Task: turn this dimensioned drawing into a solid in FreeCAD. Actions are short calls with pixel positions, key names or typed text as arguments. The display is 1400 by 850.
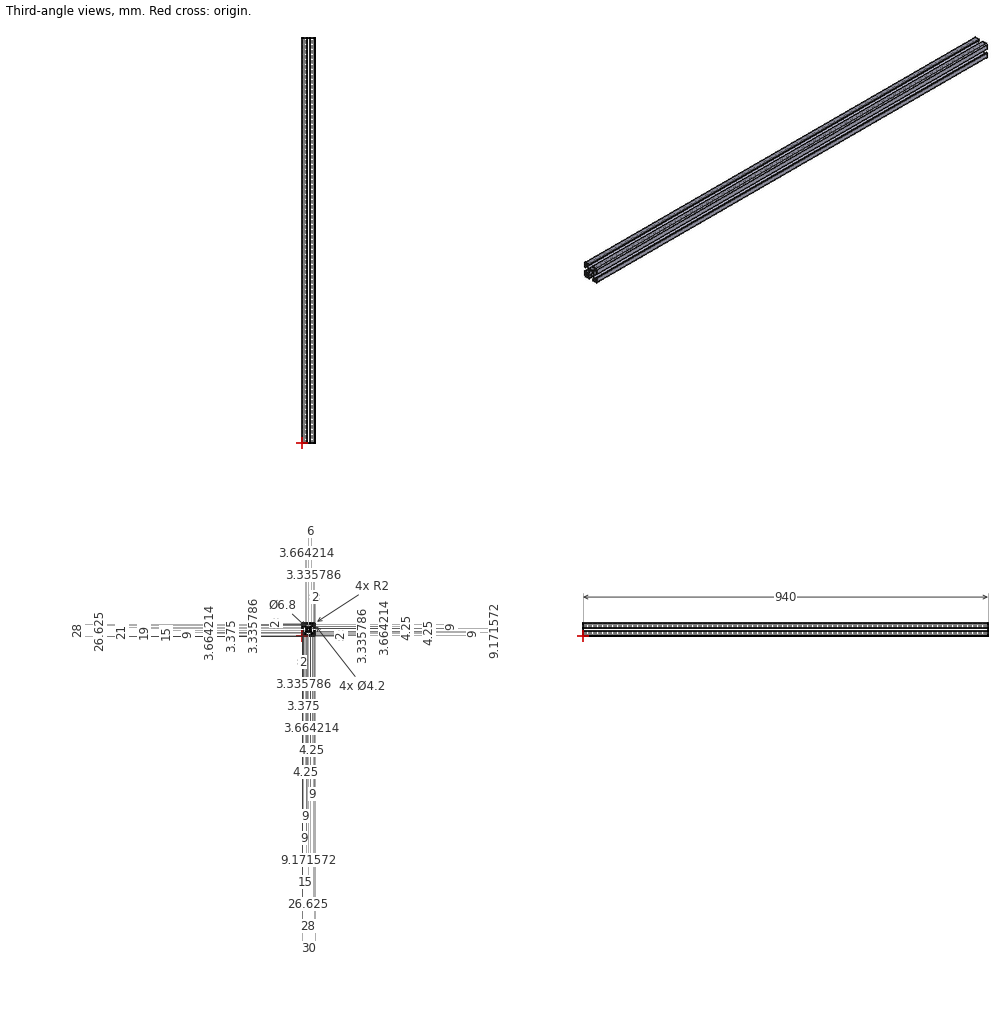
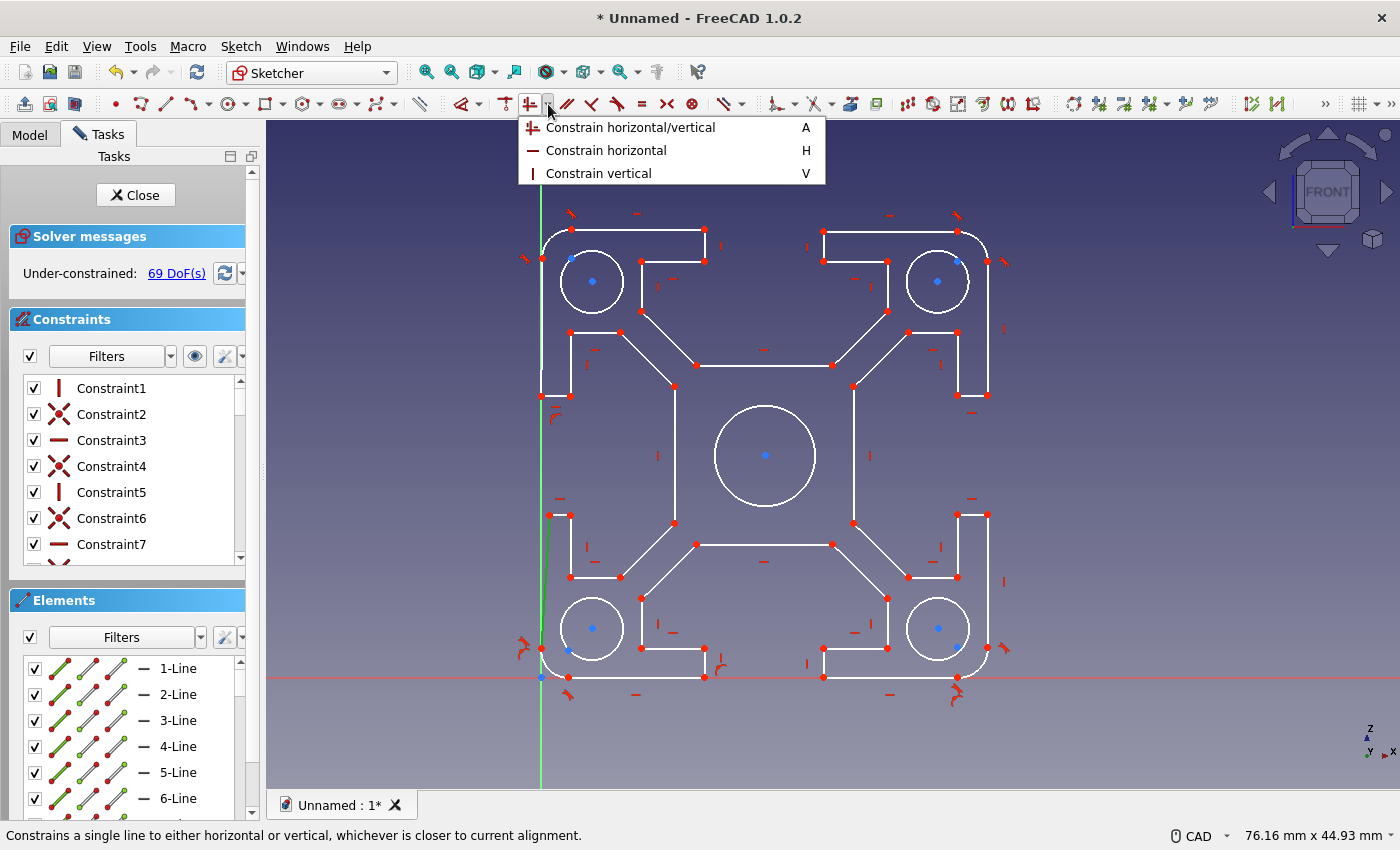
click(672, 174)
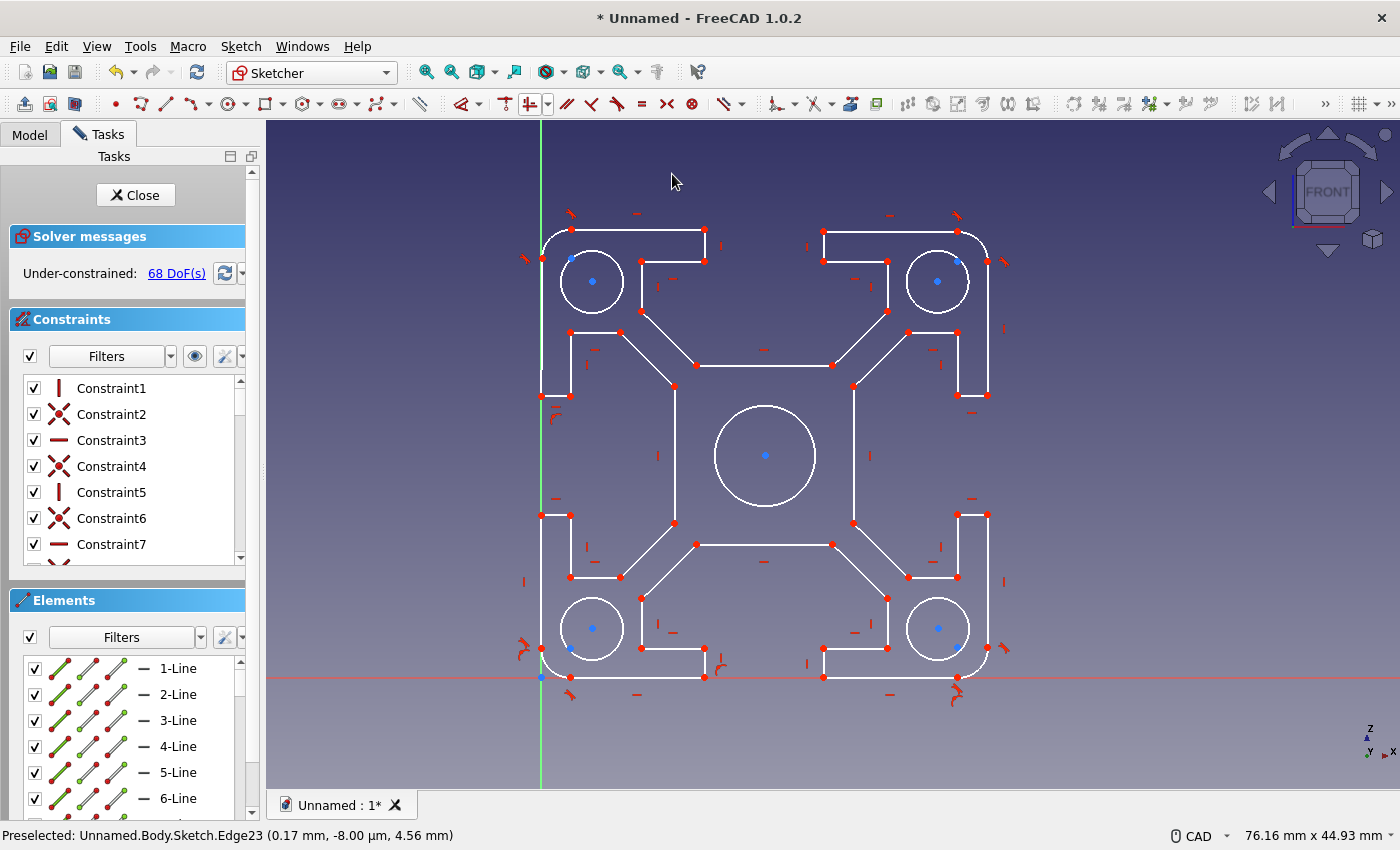
click(542, 355)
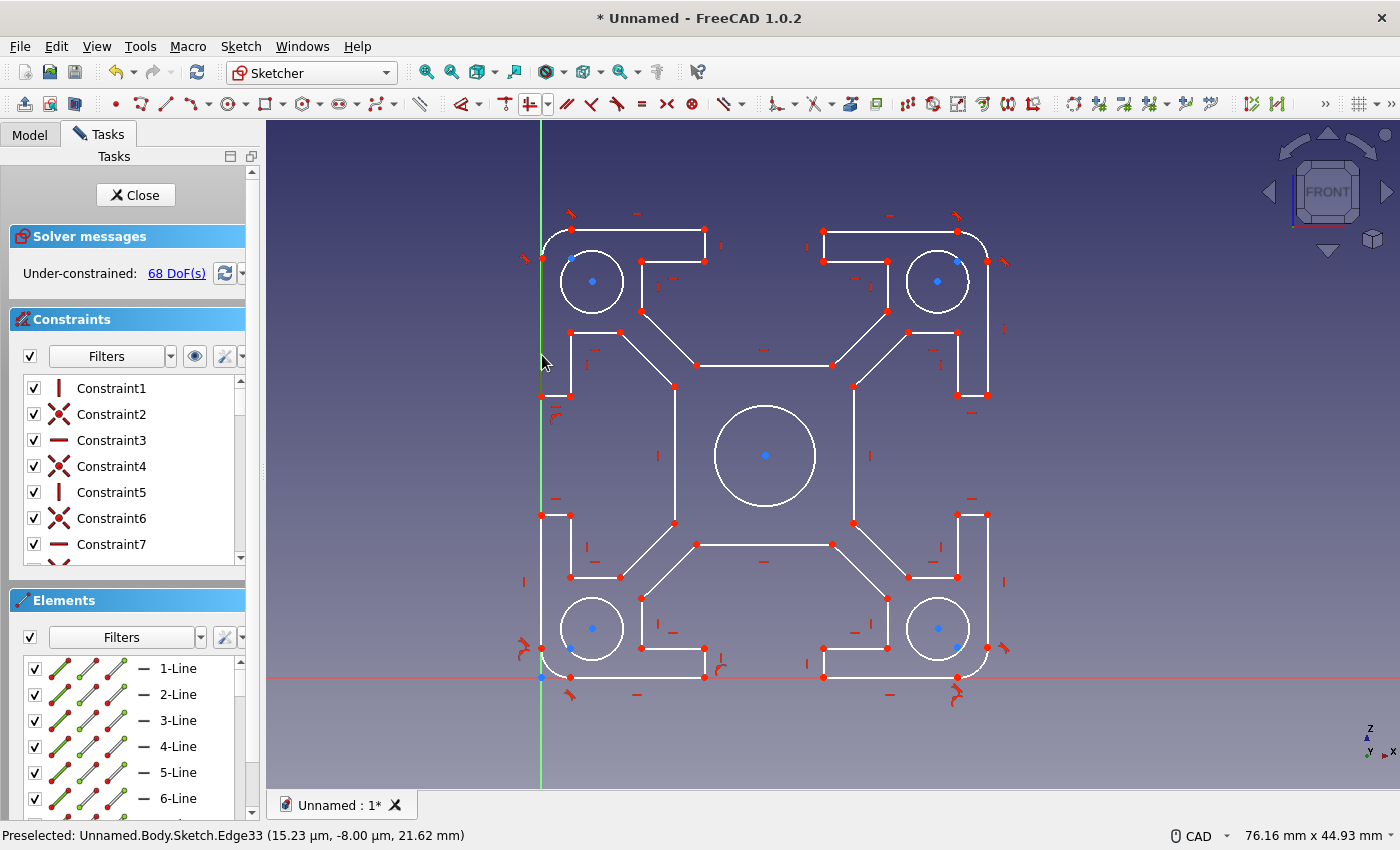
key(v)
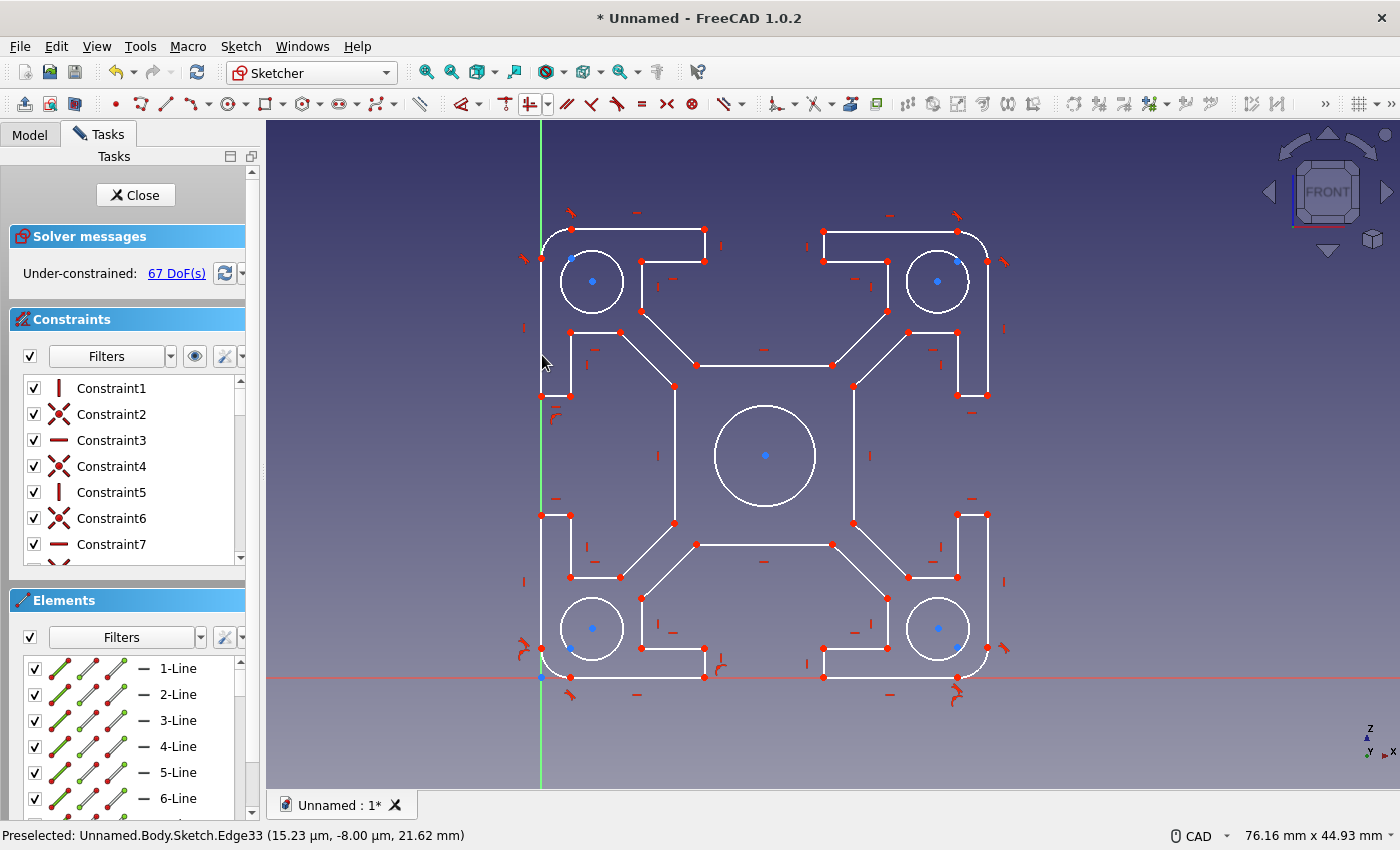
click(972, 675)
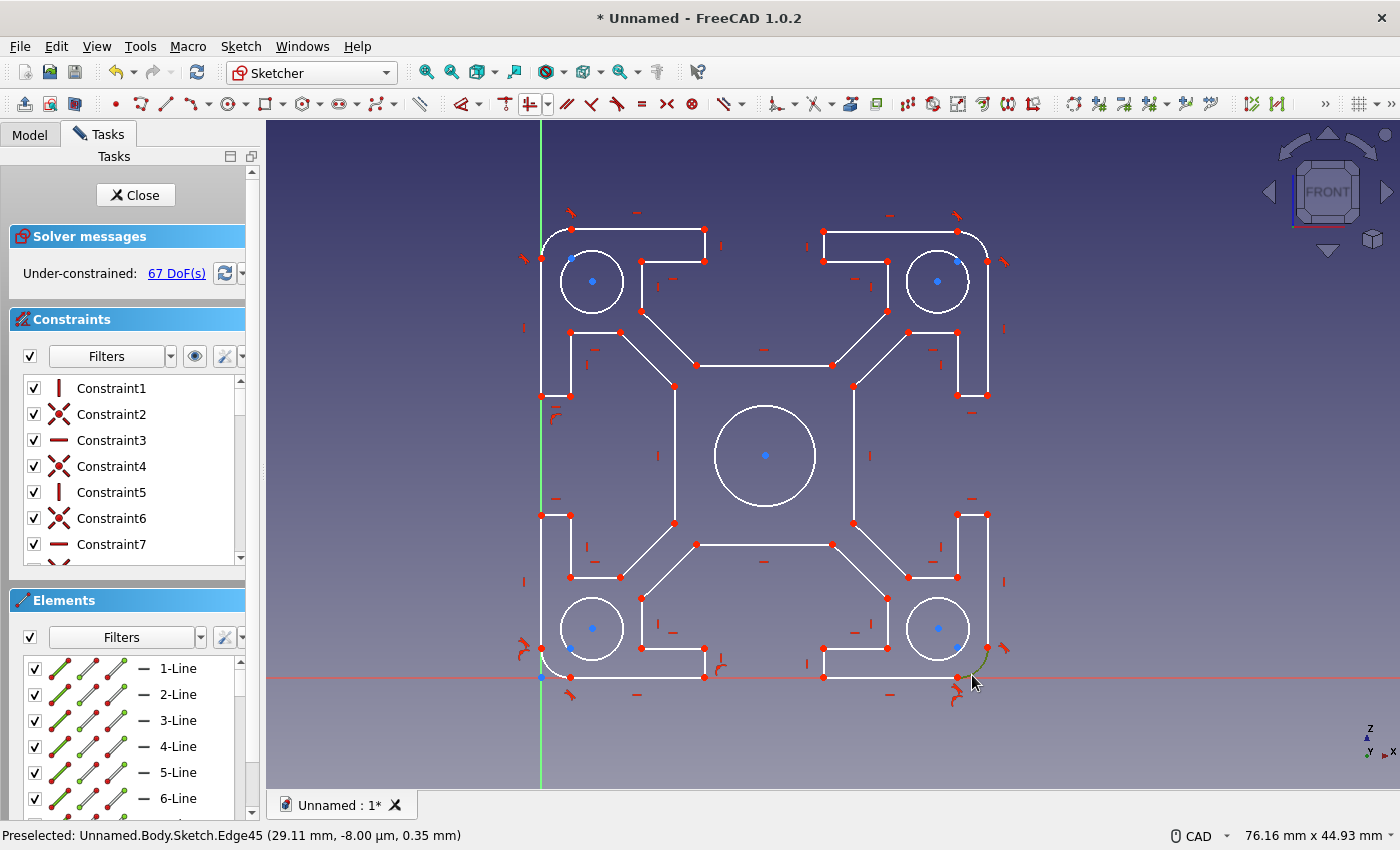
click(545, 662)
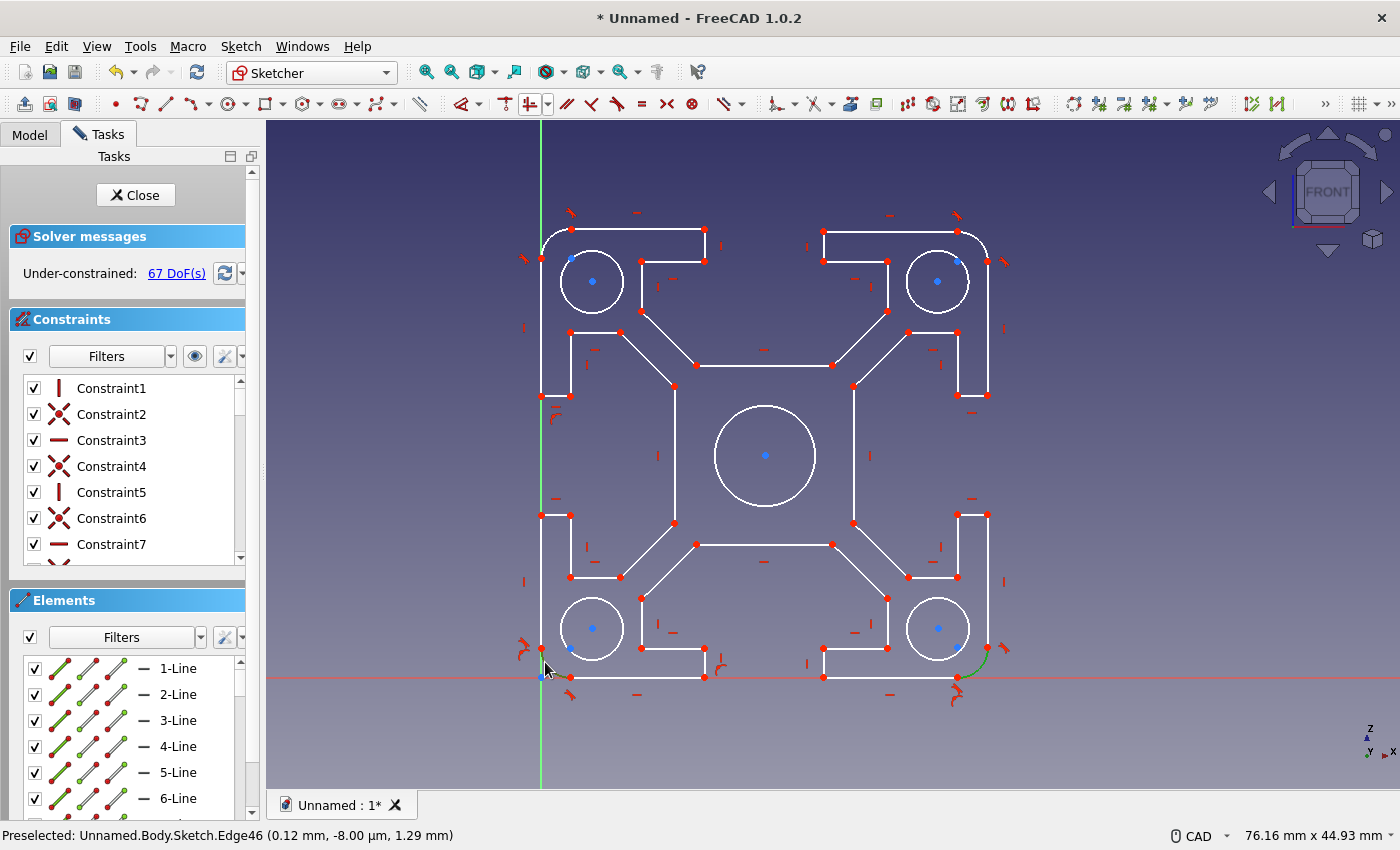
click(558, 232)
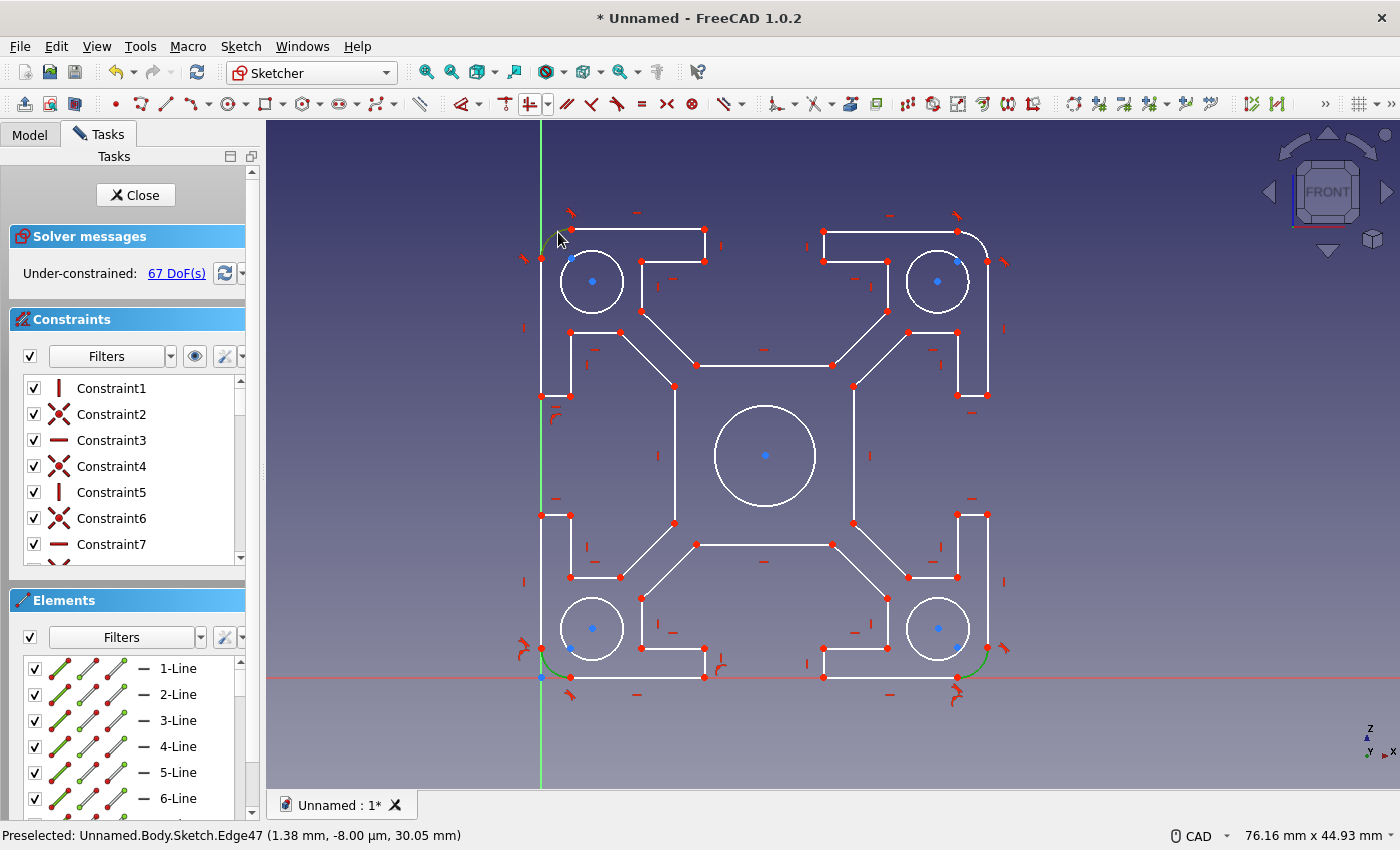
click(985, 248)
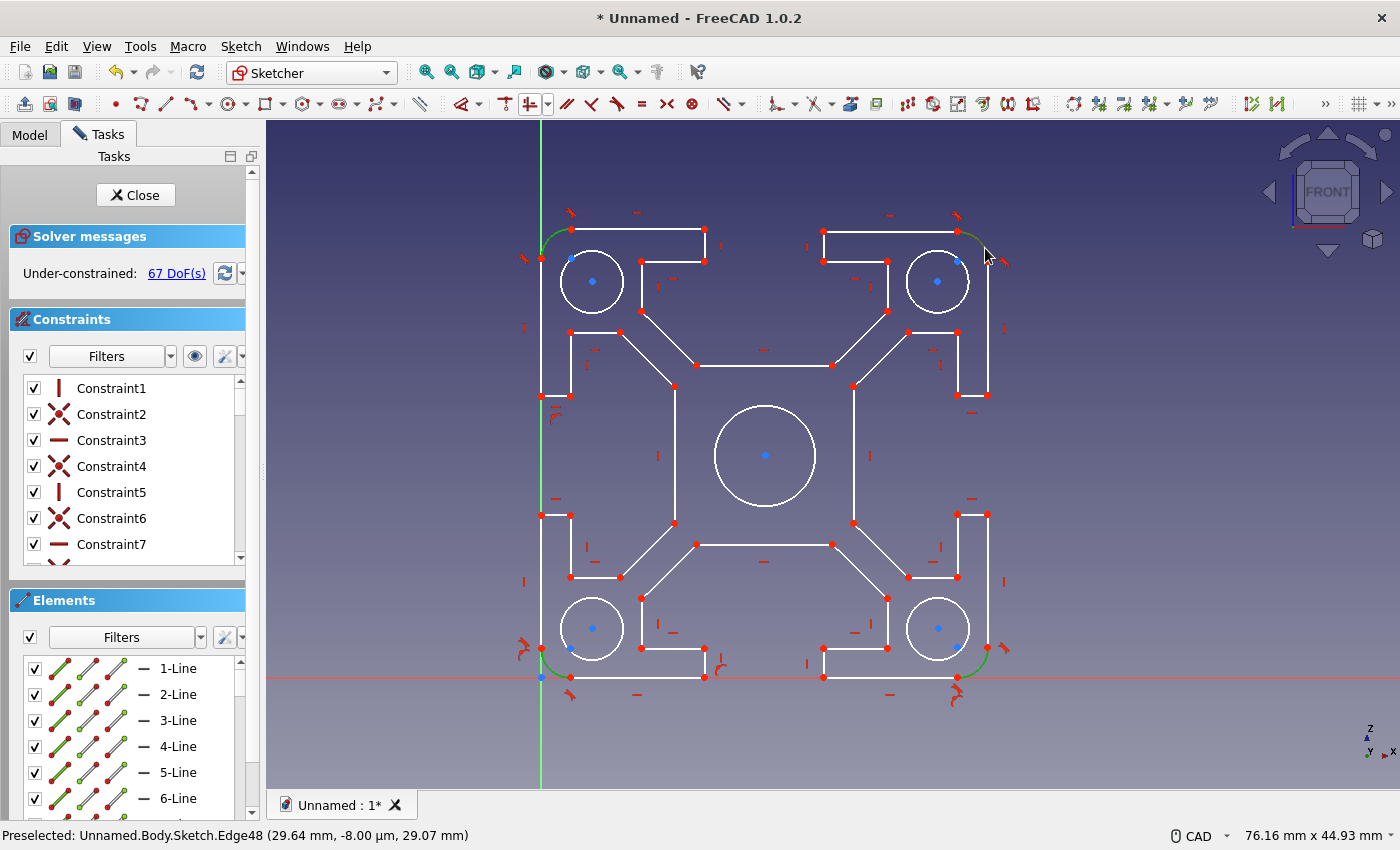
key(e)